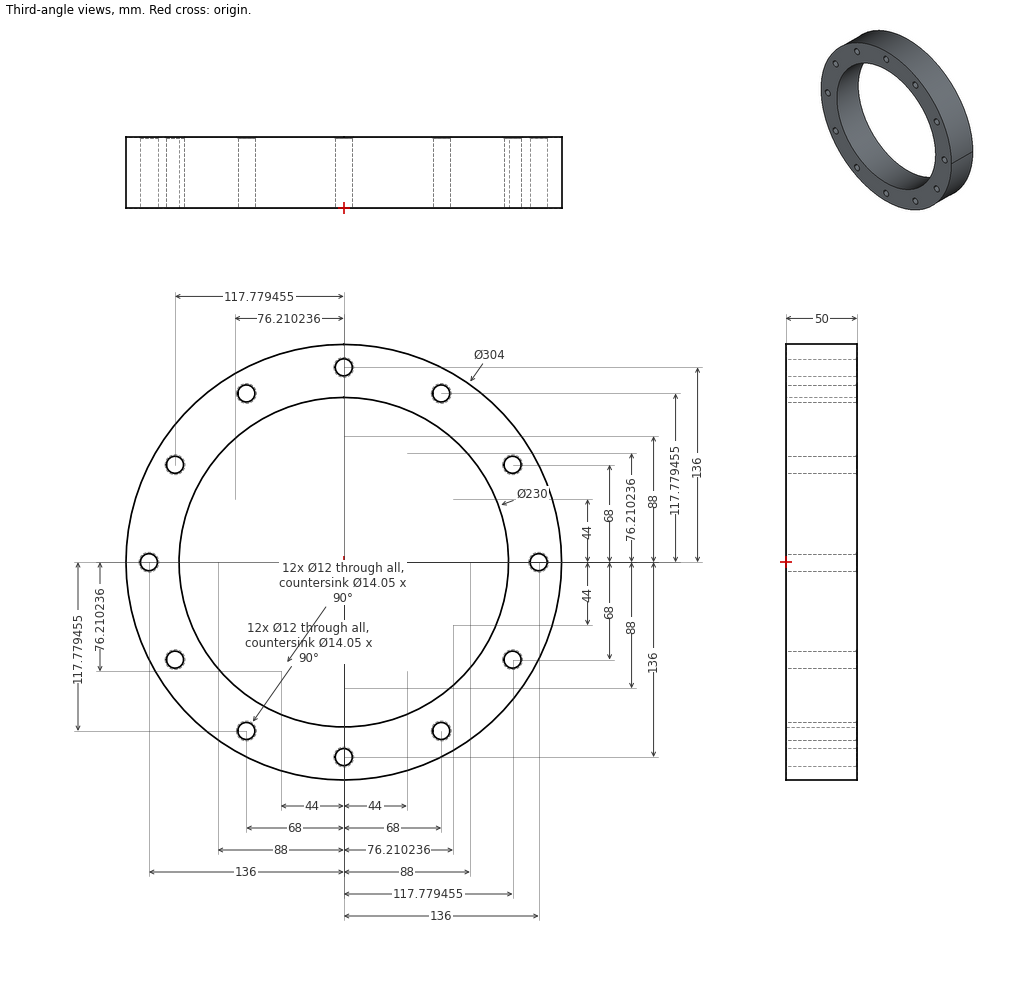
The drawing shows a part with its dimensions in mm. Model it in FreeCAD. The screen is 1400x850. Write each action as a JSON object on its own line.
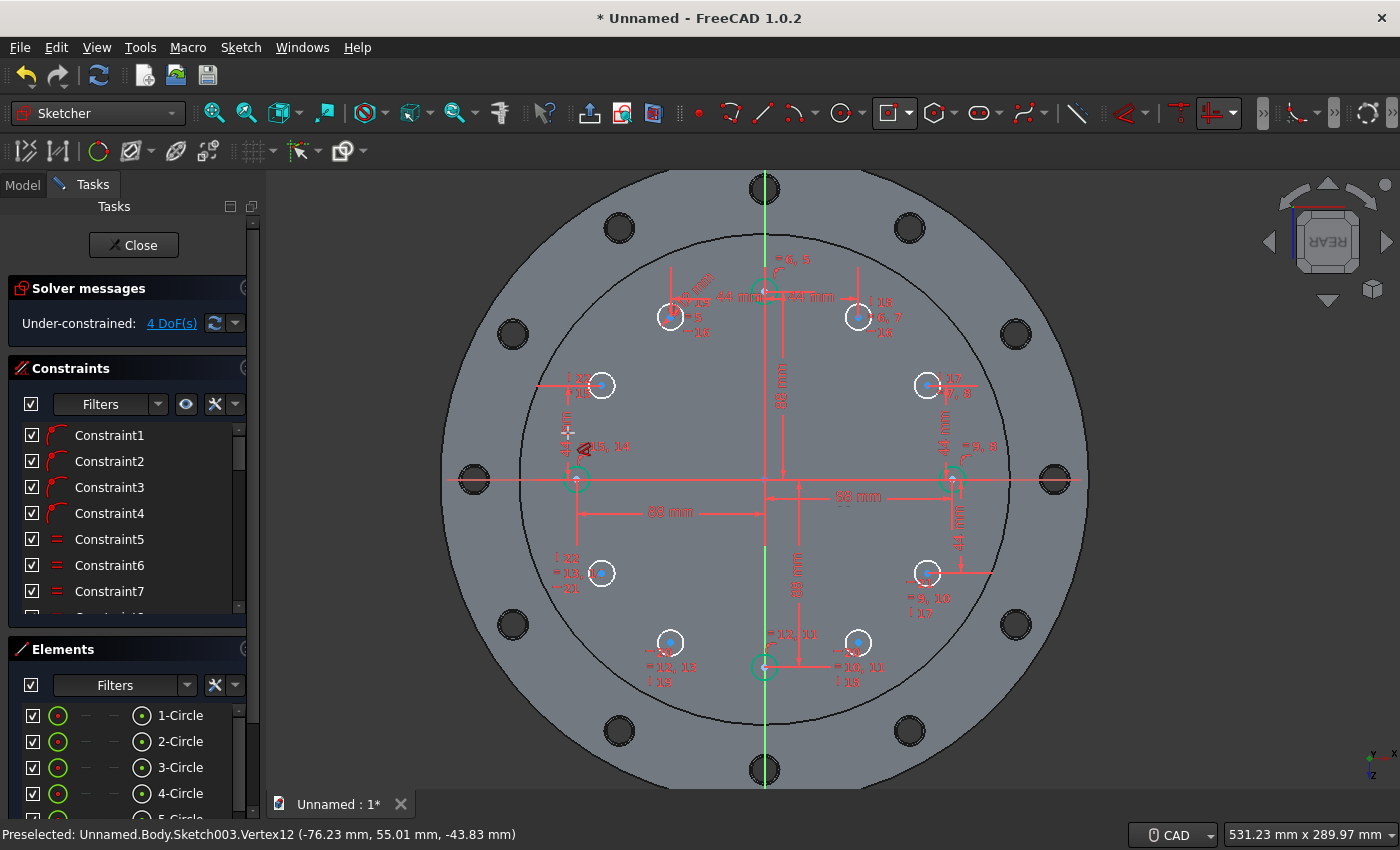
{"action": "left_click", "coordinate": [671, 317]}
{"action": "left_click", "coordinate": [637, 398]}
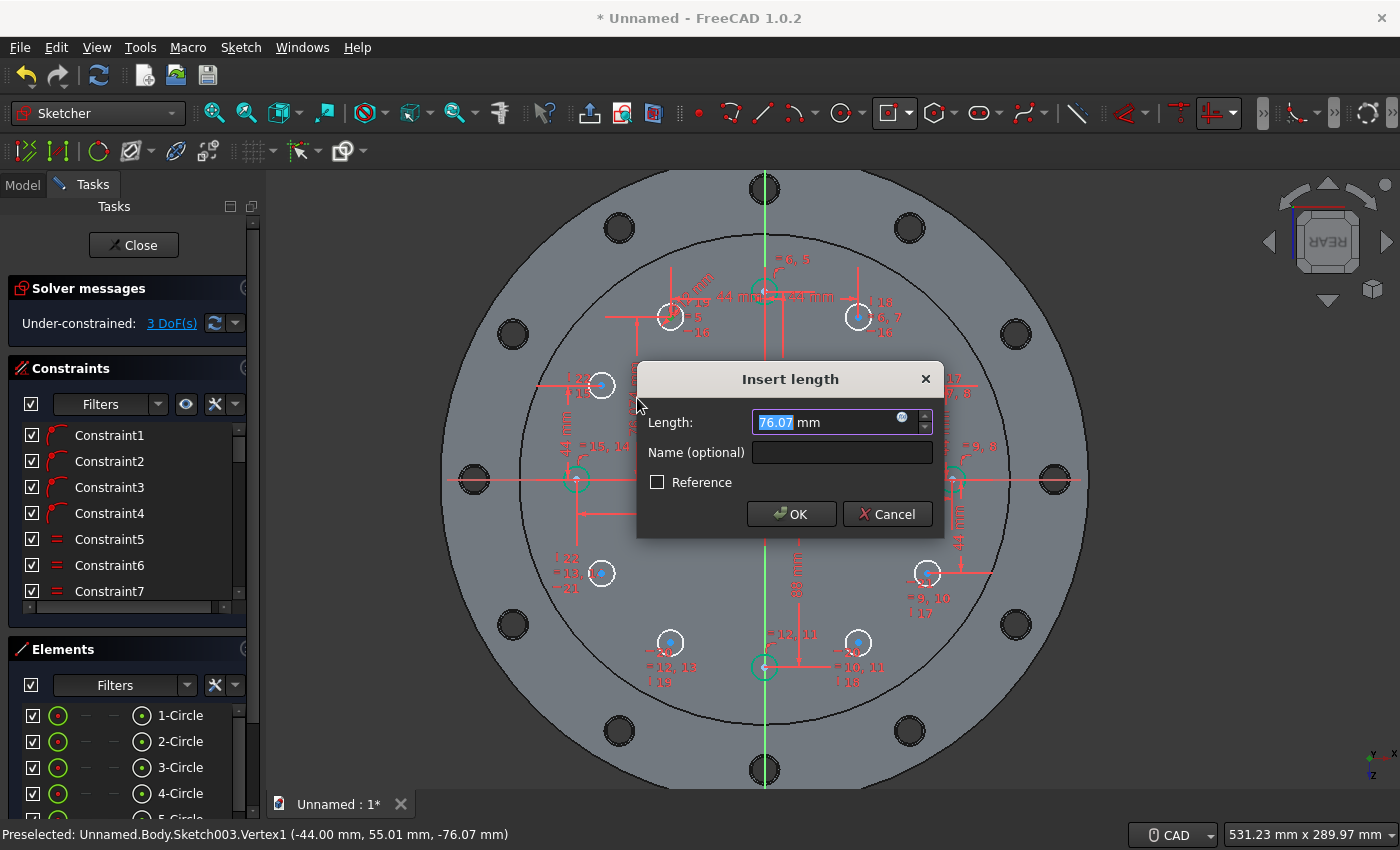
{"action": "type", "text": "76.210236"}
{"action": "key", "text": "Return"}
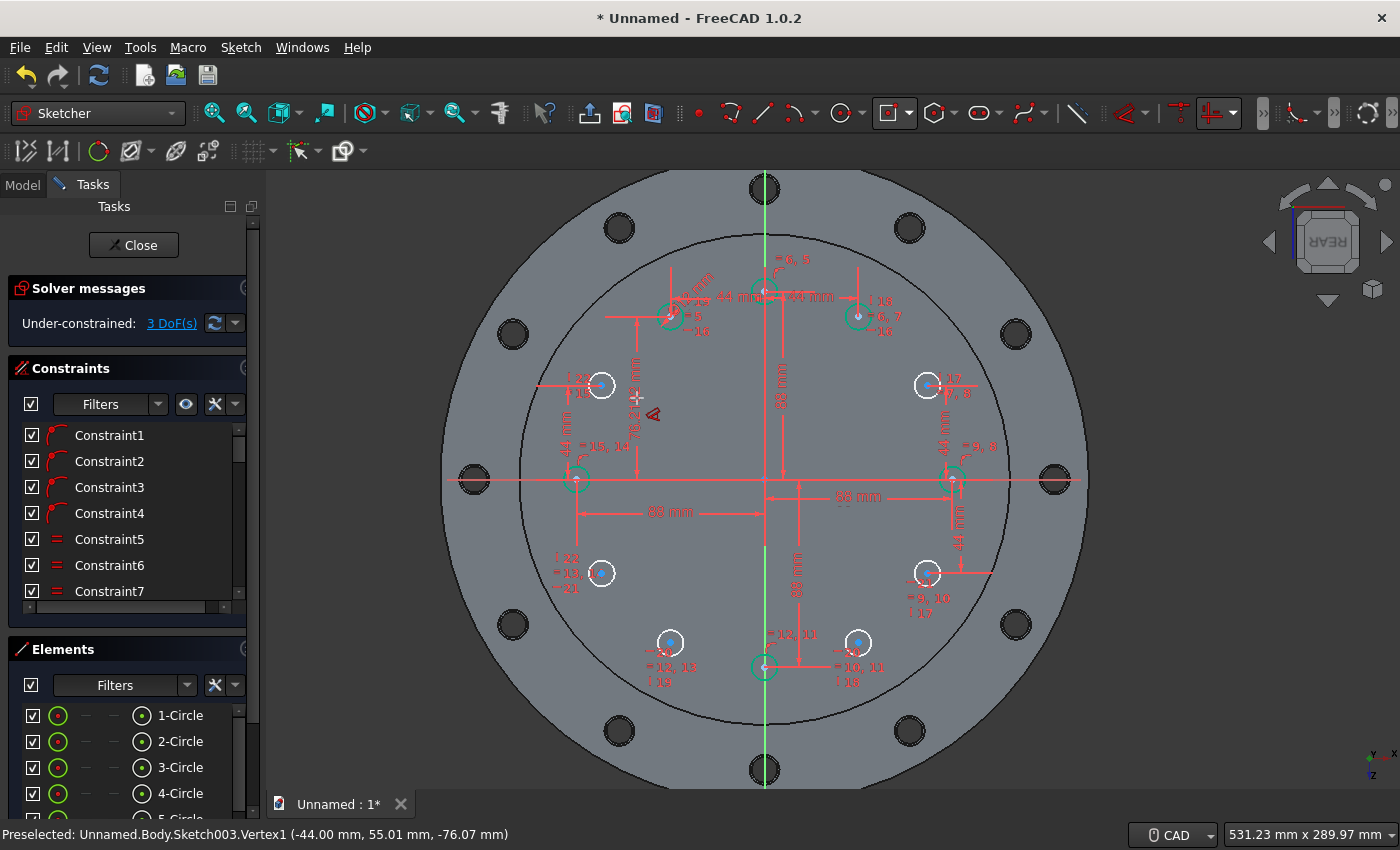
{"action": "left_click", "coordinate": [927, 386]}
{"action": "left_click", "coordinate": [846, 352]}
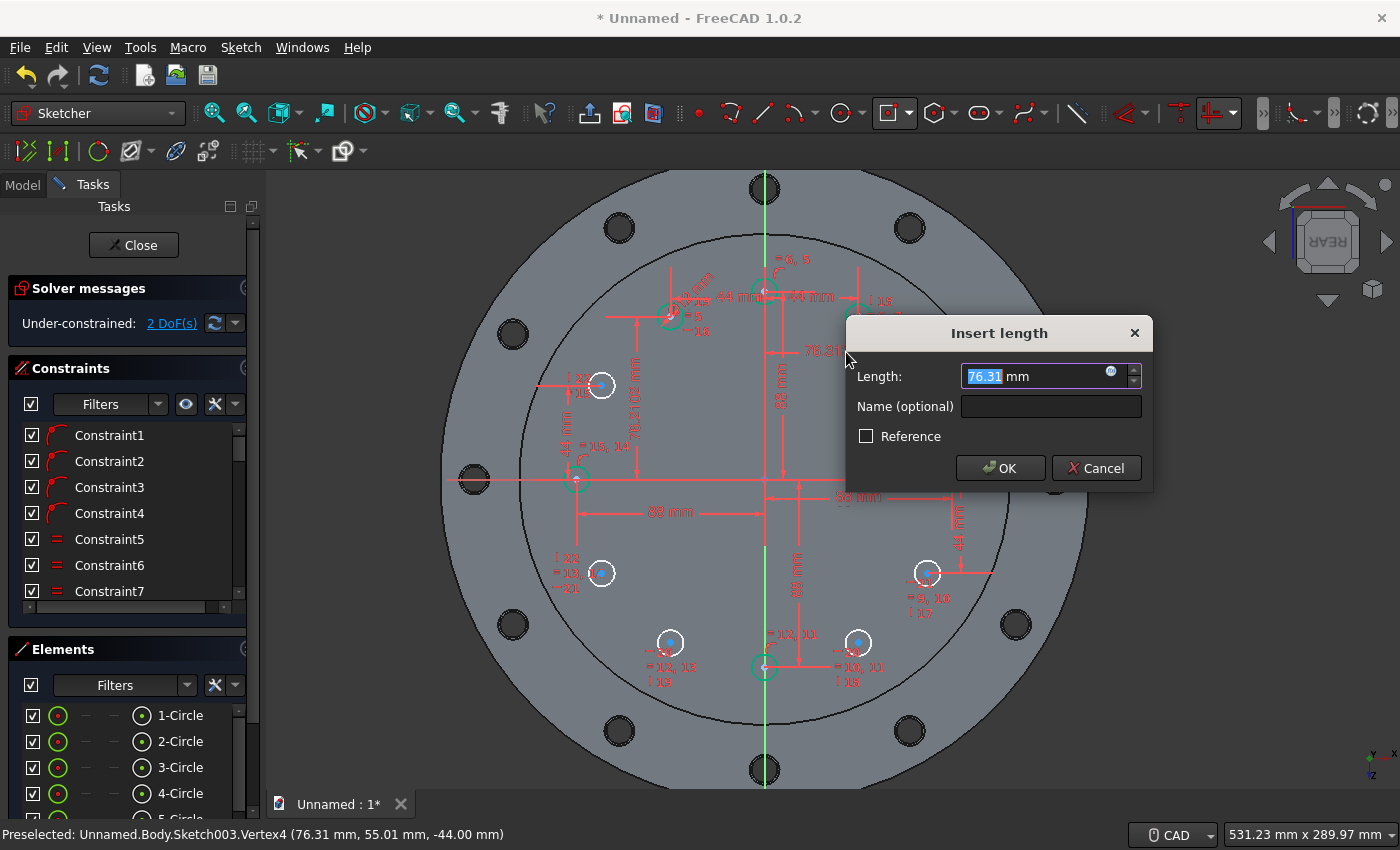
{"action": "type", "text": "76.210236"}
{"action": "key", "text": "Return"}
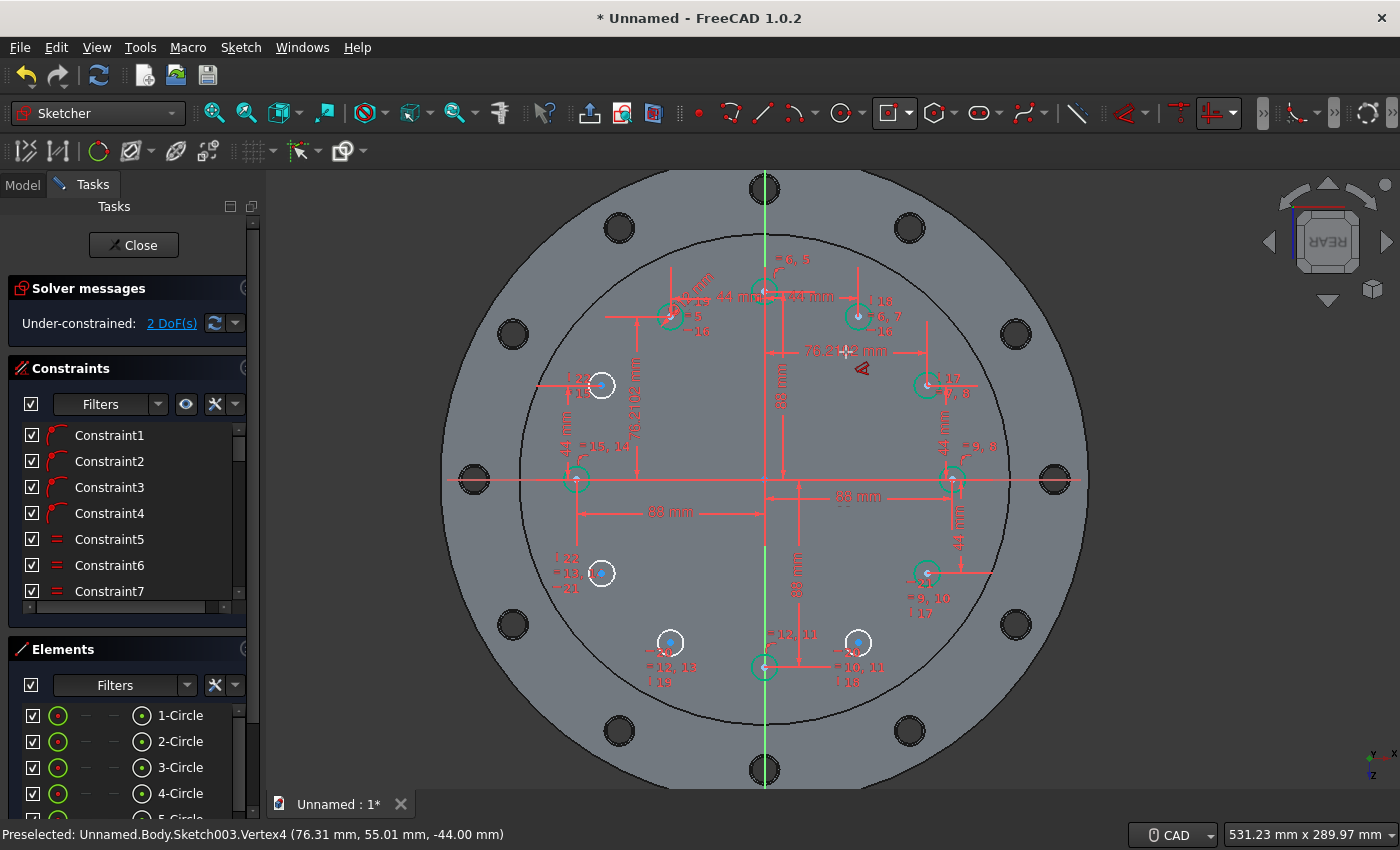
{"action": "left_click", "coordinate": [858, 643]}
{"action": "left_click", "coordinate": [892, 561]}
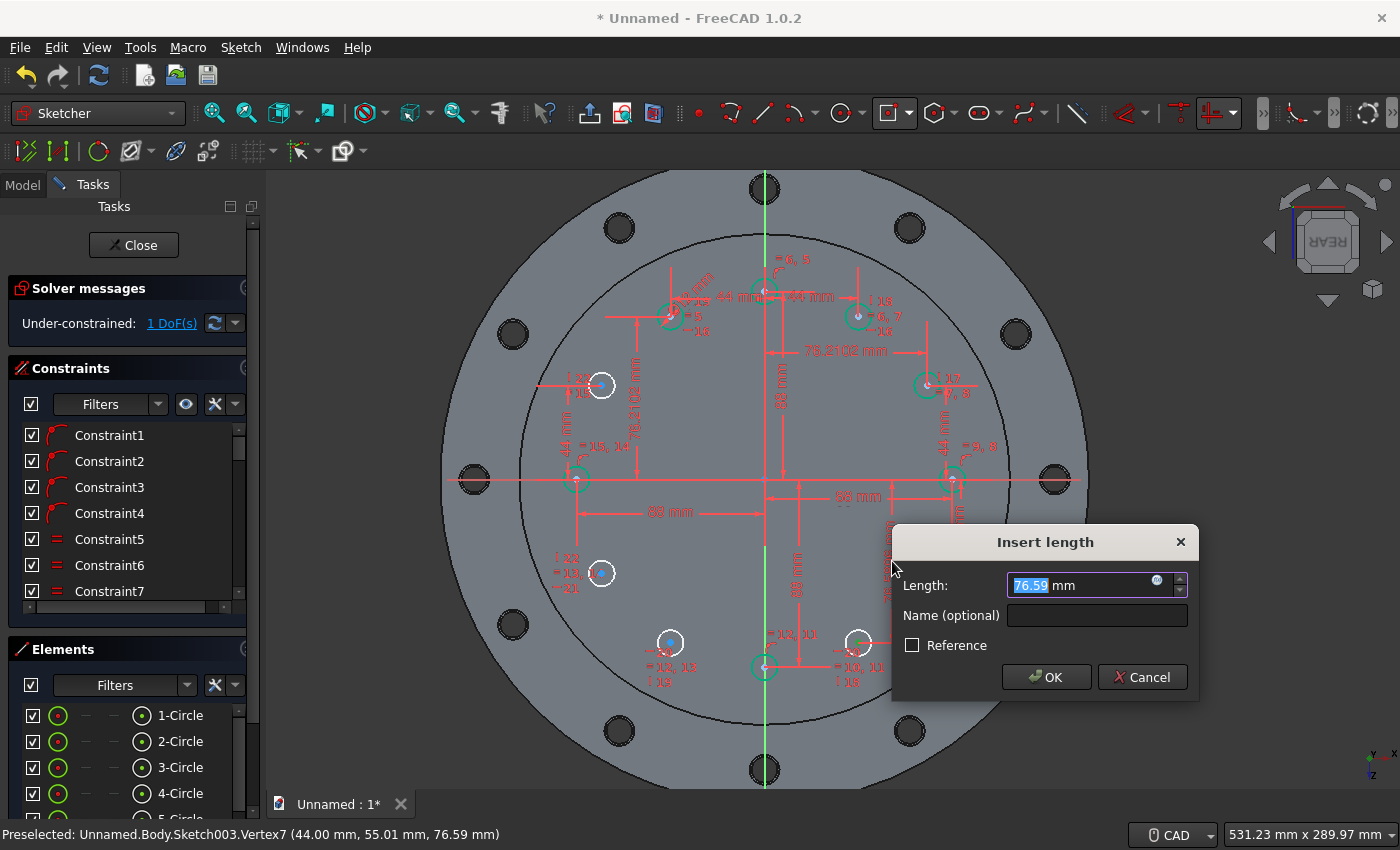
{"action": "type", "text": "76.210236"}
{"action": "key", "text": "Return"}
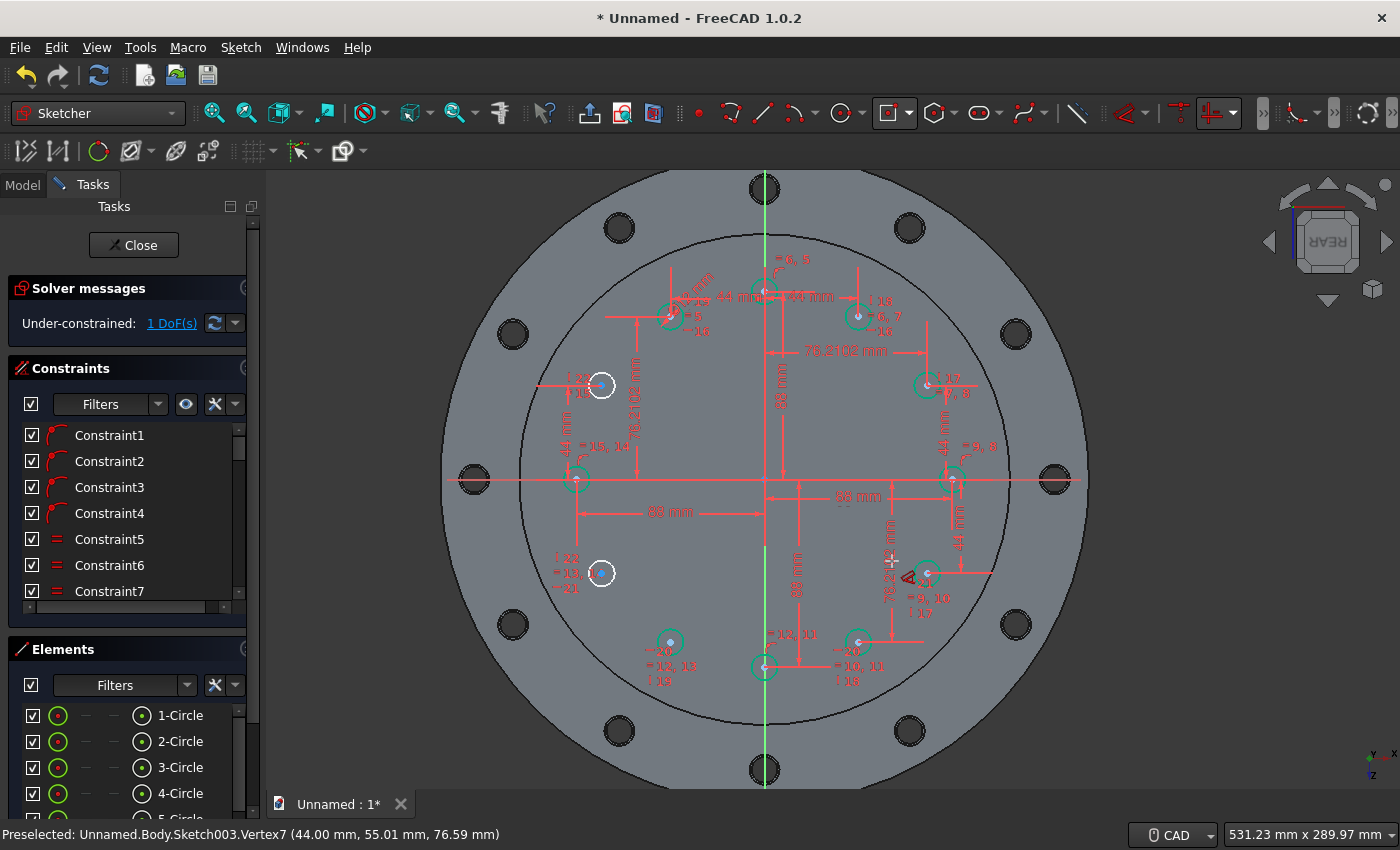
{"action": "left_click", "coordinate": [602, 573]}
{"action": "left_click", "coordinate": [683, 607]}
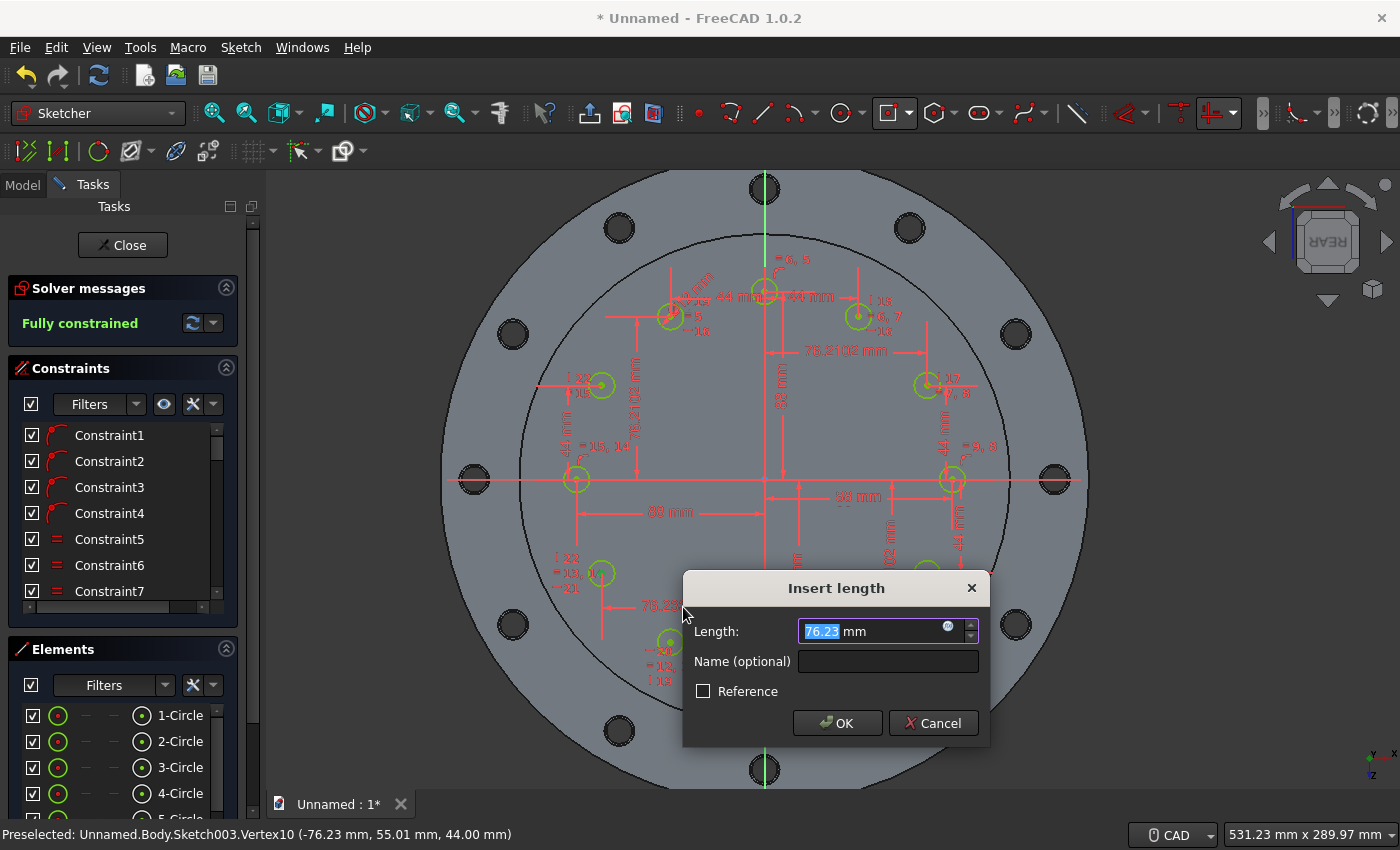
{"action": "type", "text": "76.210236"}
{"action": "key", "text": "Return"}
{"action": "key", "text": "Escape"}